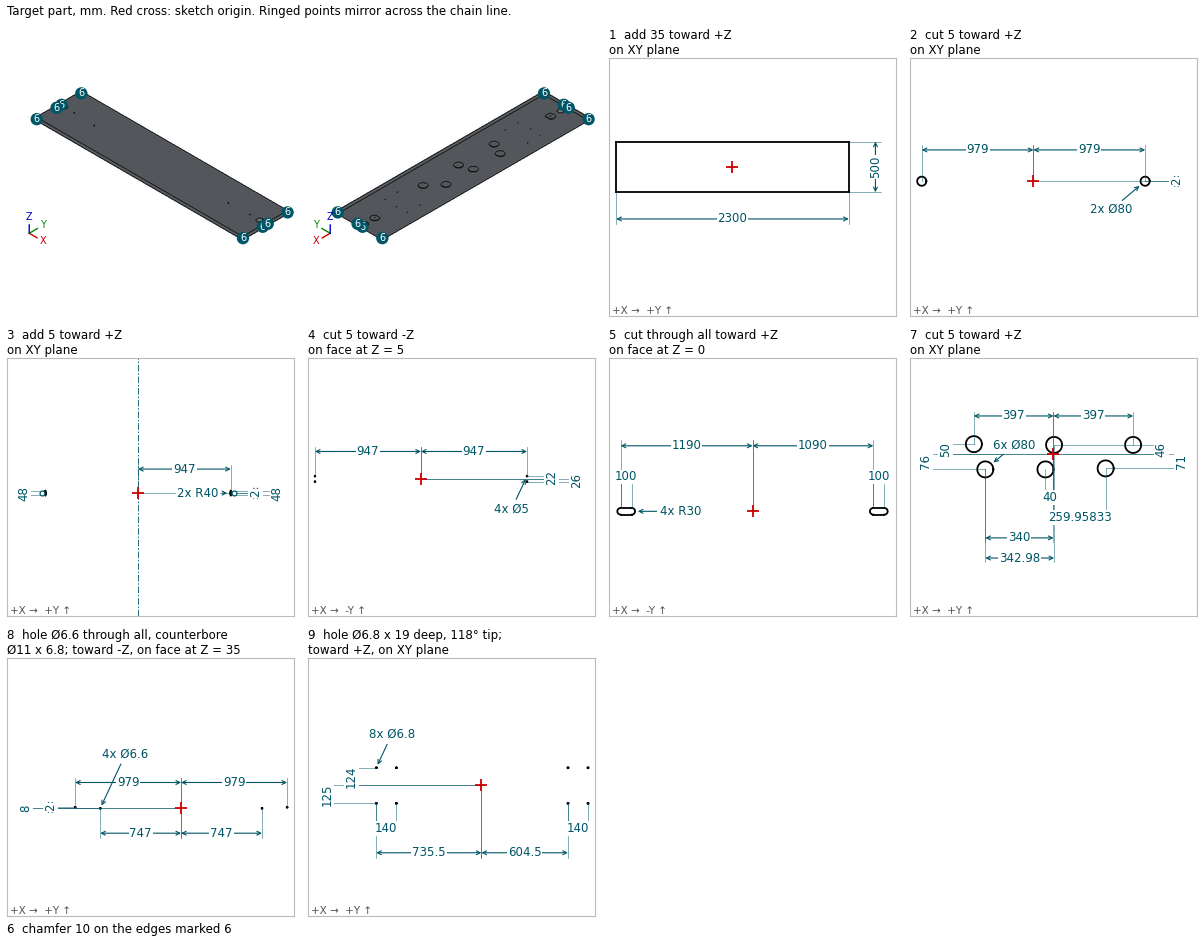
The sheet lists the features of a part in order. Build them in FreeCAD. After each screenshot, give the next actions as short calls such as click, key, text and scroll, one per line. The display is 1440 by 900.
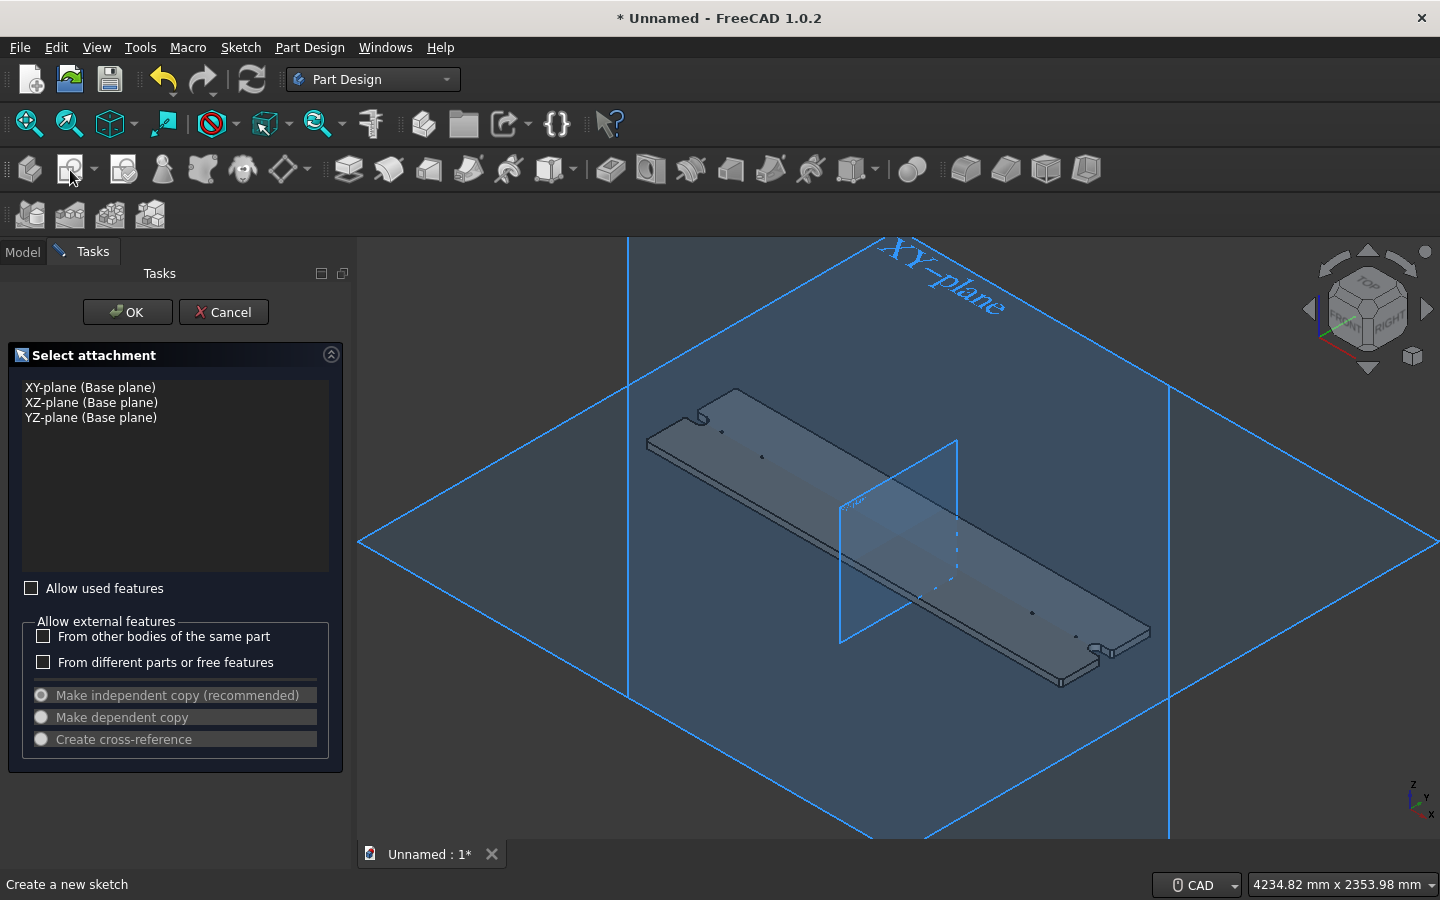
click(82, 388)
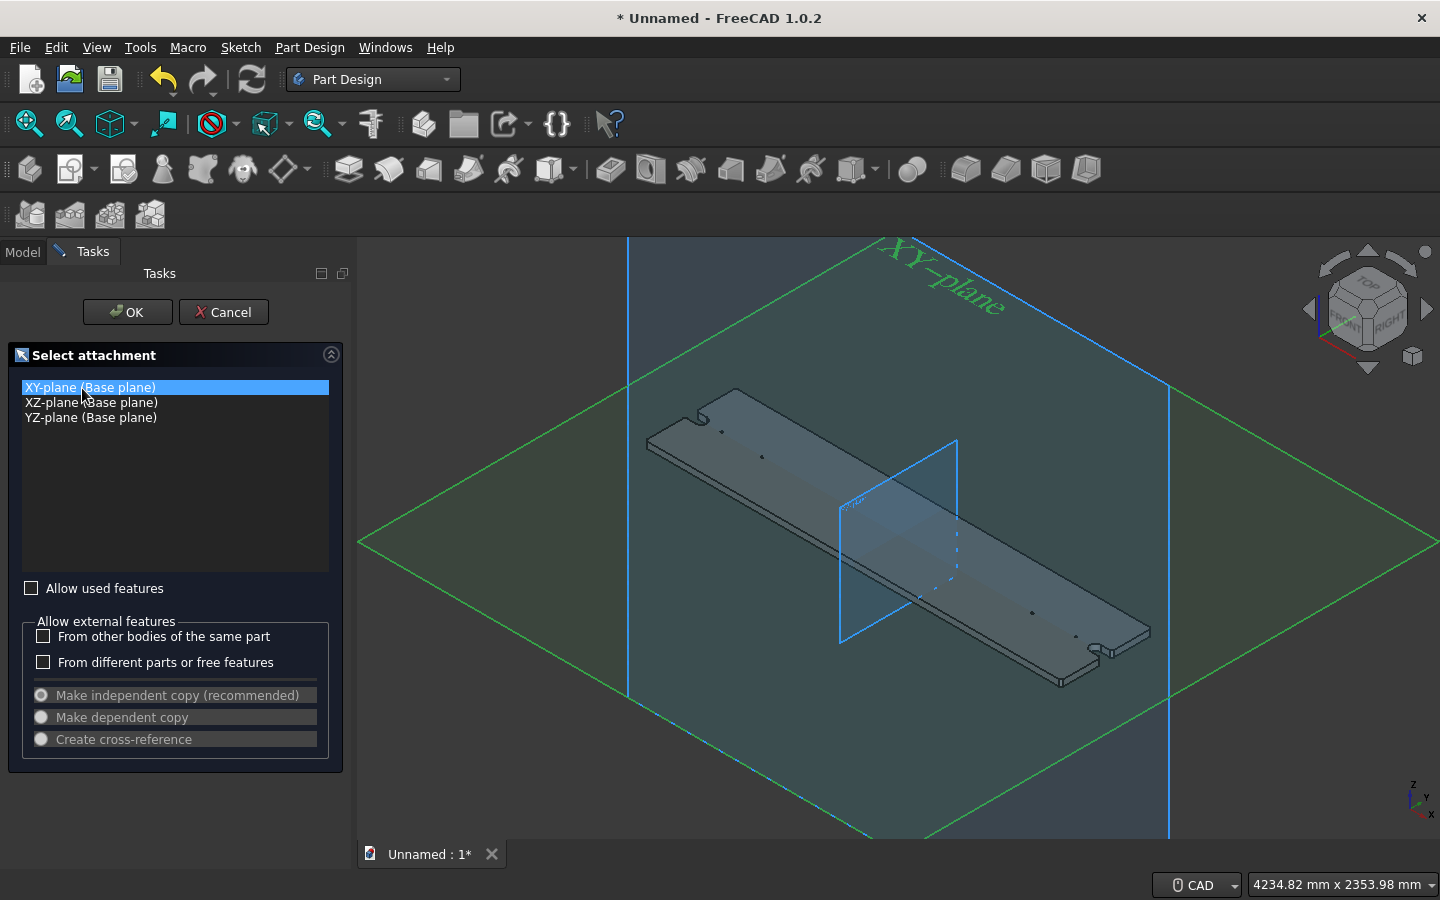
click(128, 312)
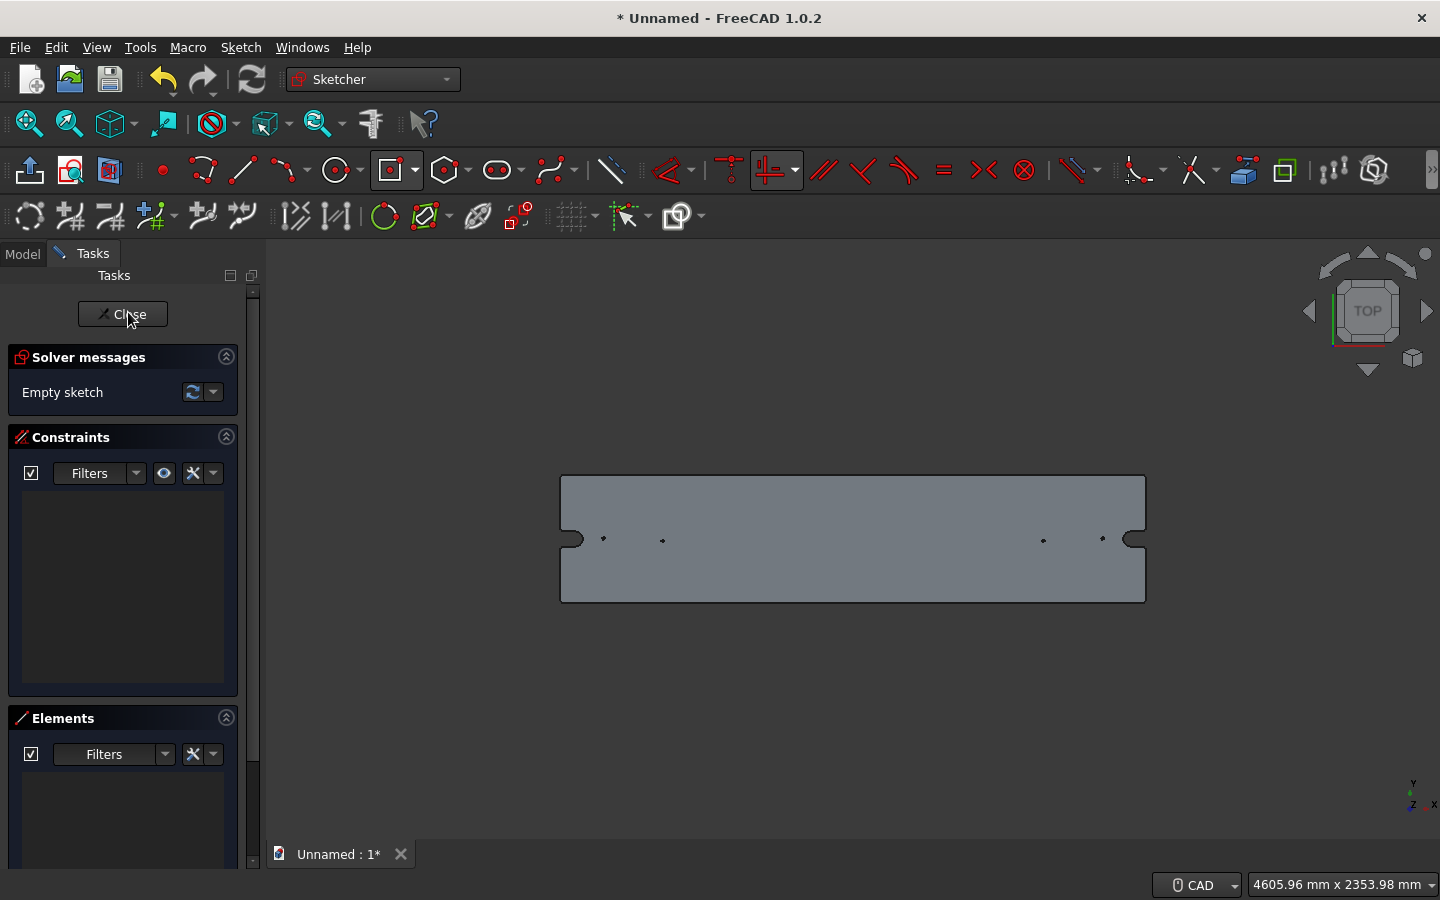
key(q)
key(s)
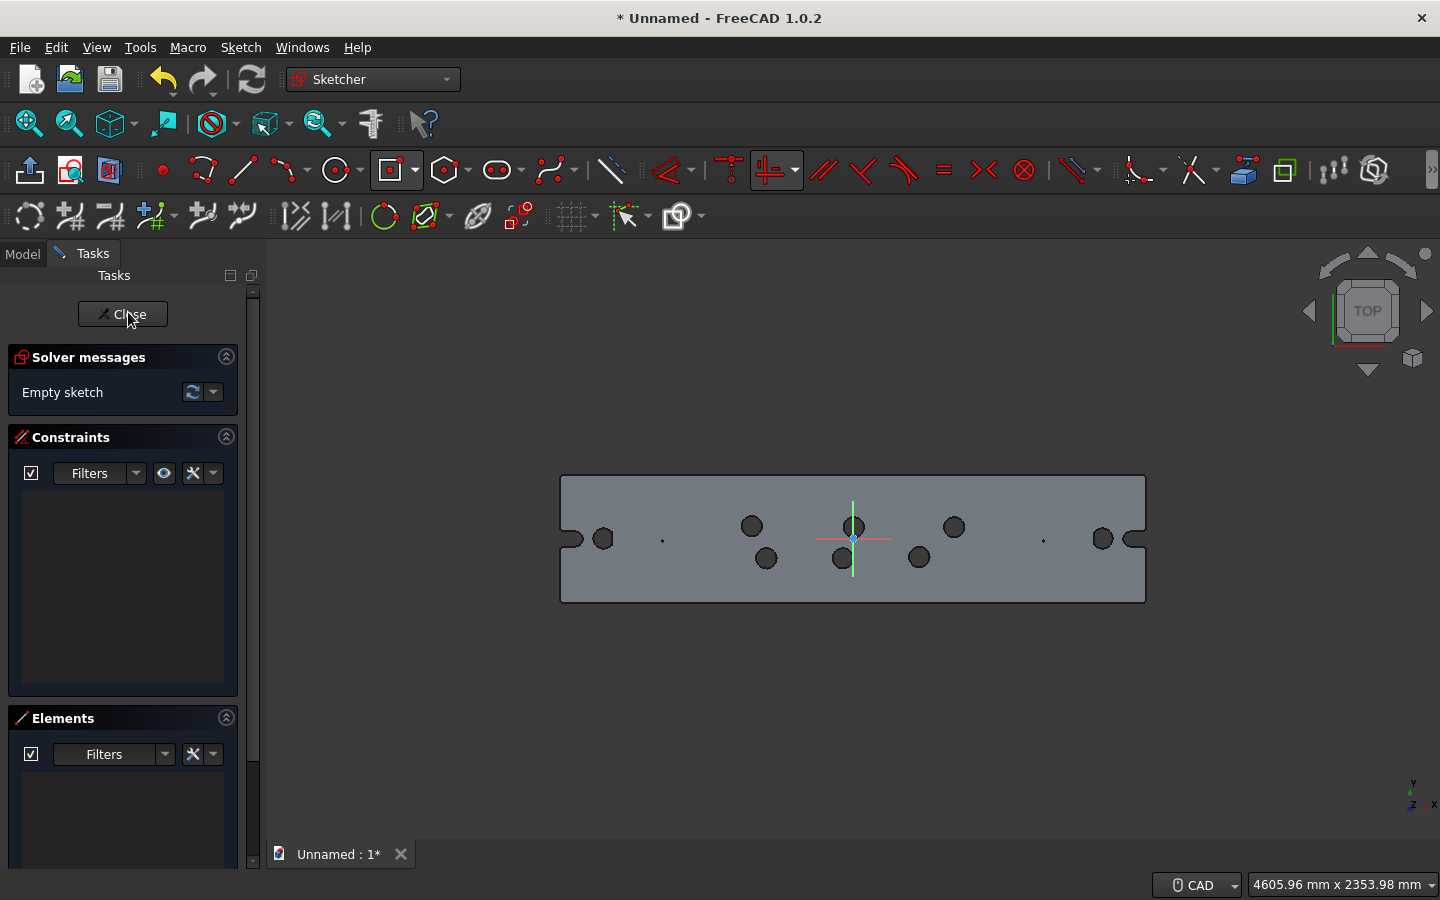
scroll(939, 539, up, 3)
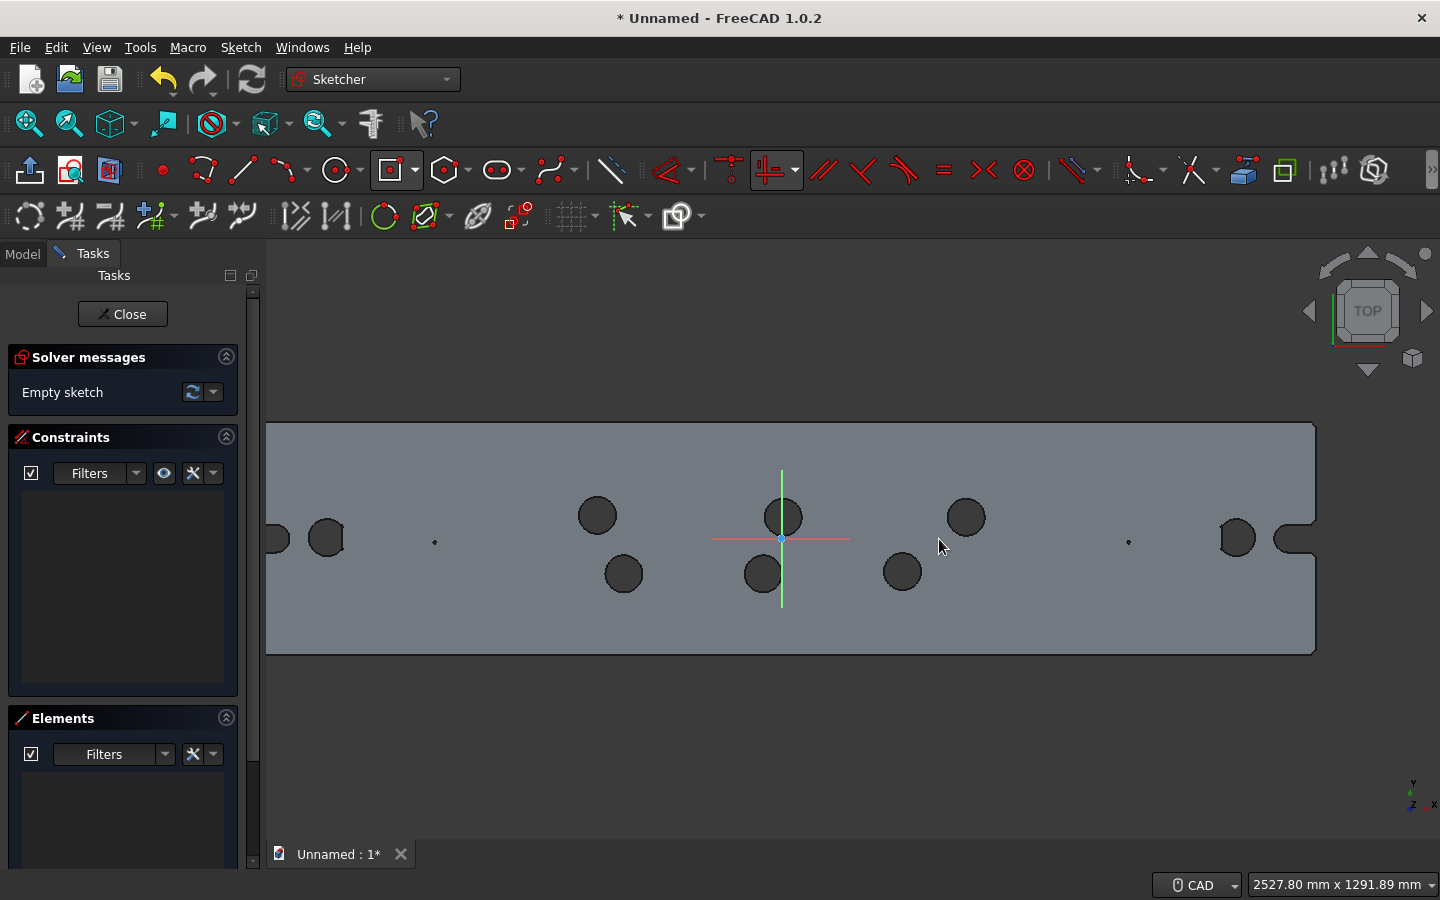
click(336, 170)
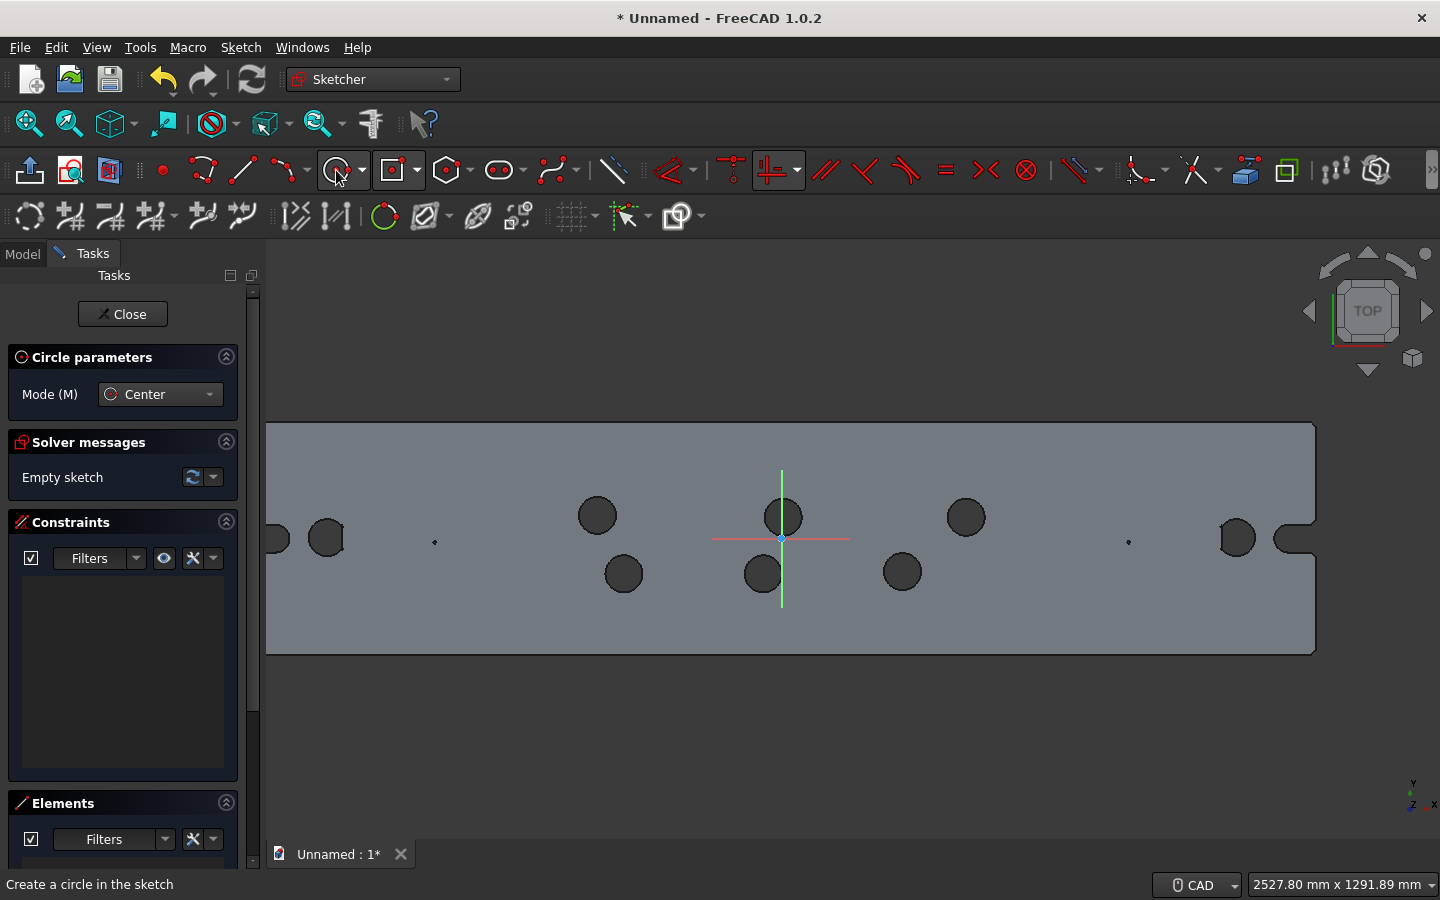
scroll(440, 597, up, 14)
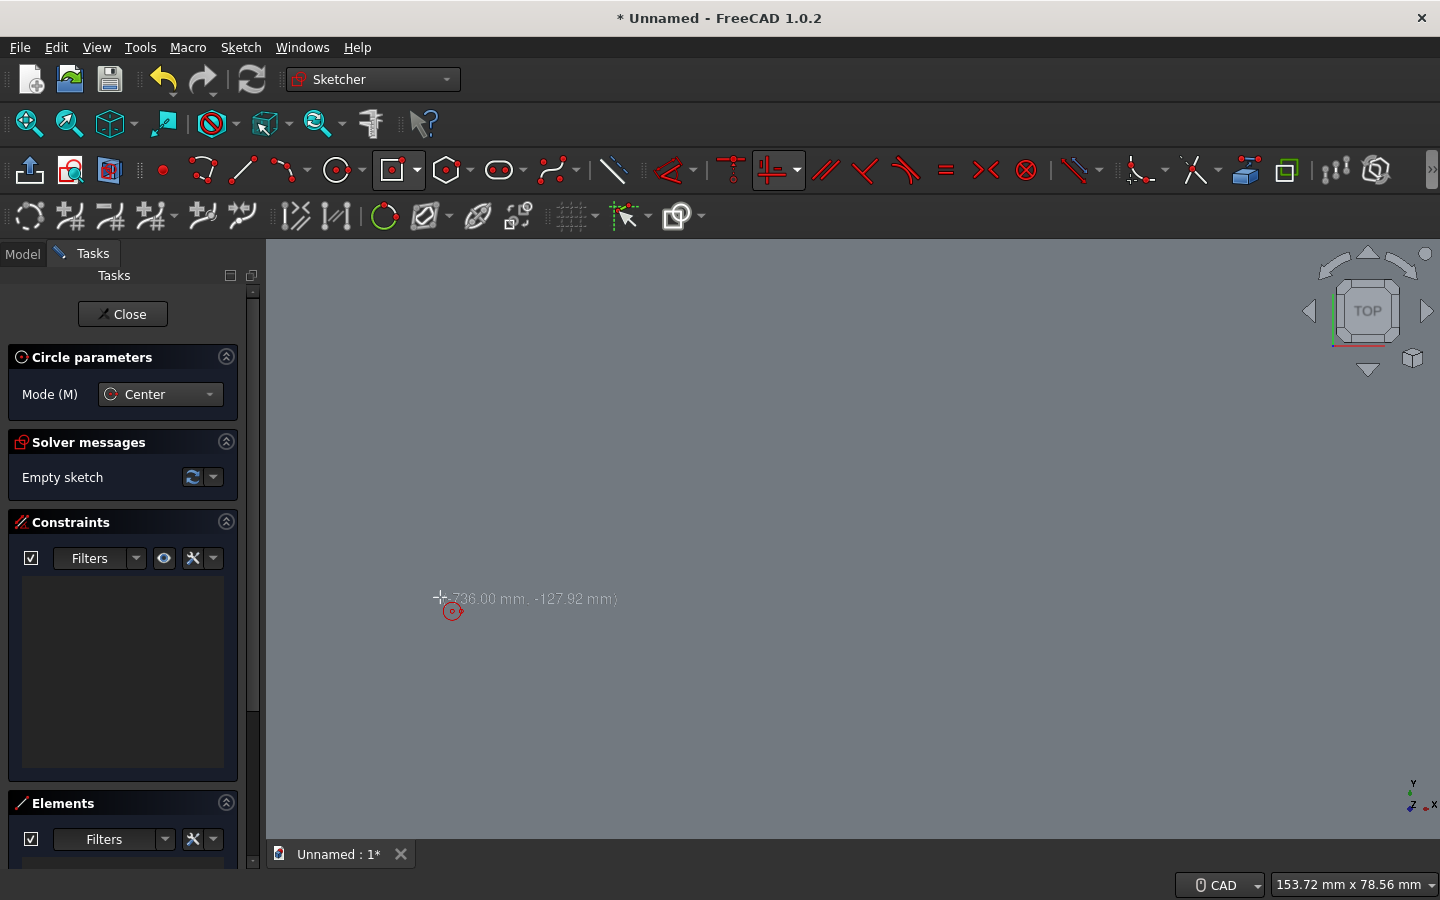
scroll(441, 598, down, 14)